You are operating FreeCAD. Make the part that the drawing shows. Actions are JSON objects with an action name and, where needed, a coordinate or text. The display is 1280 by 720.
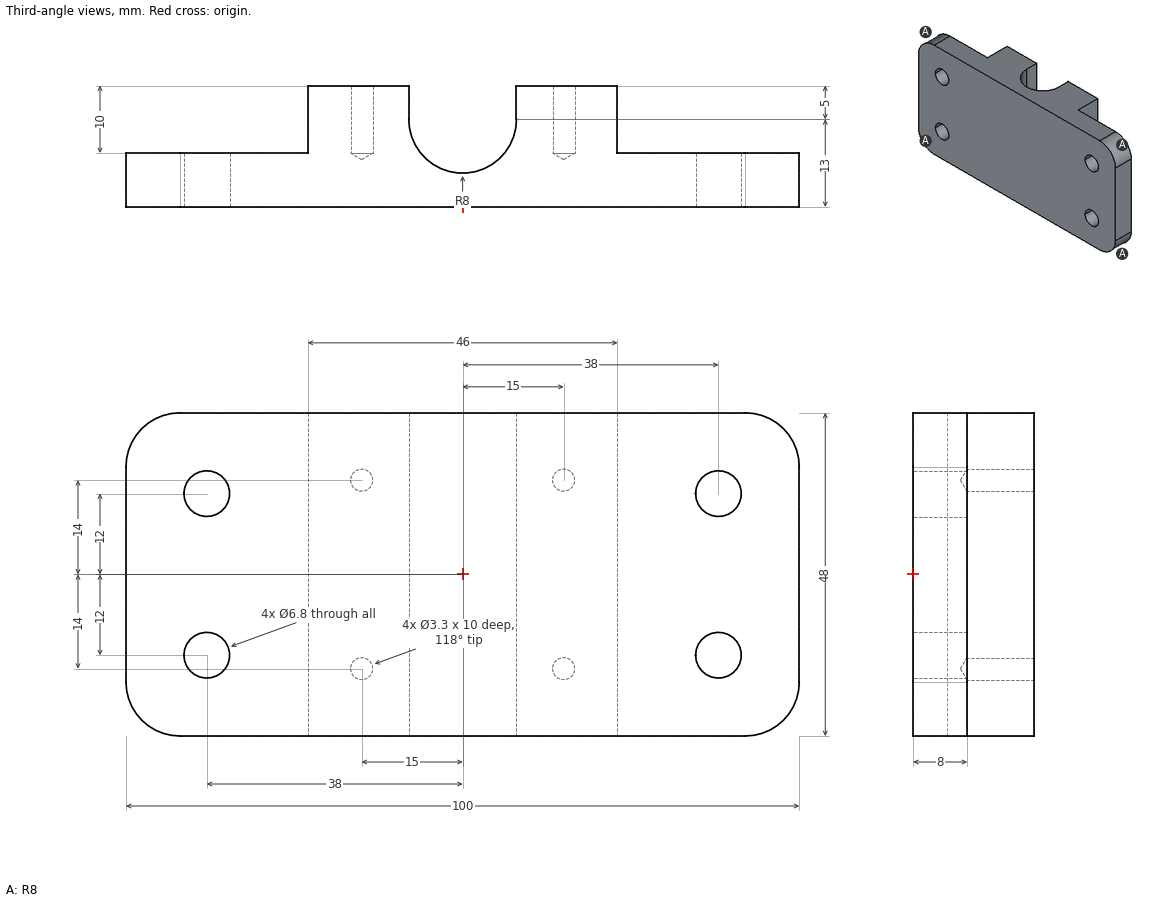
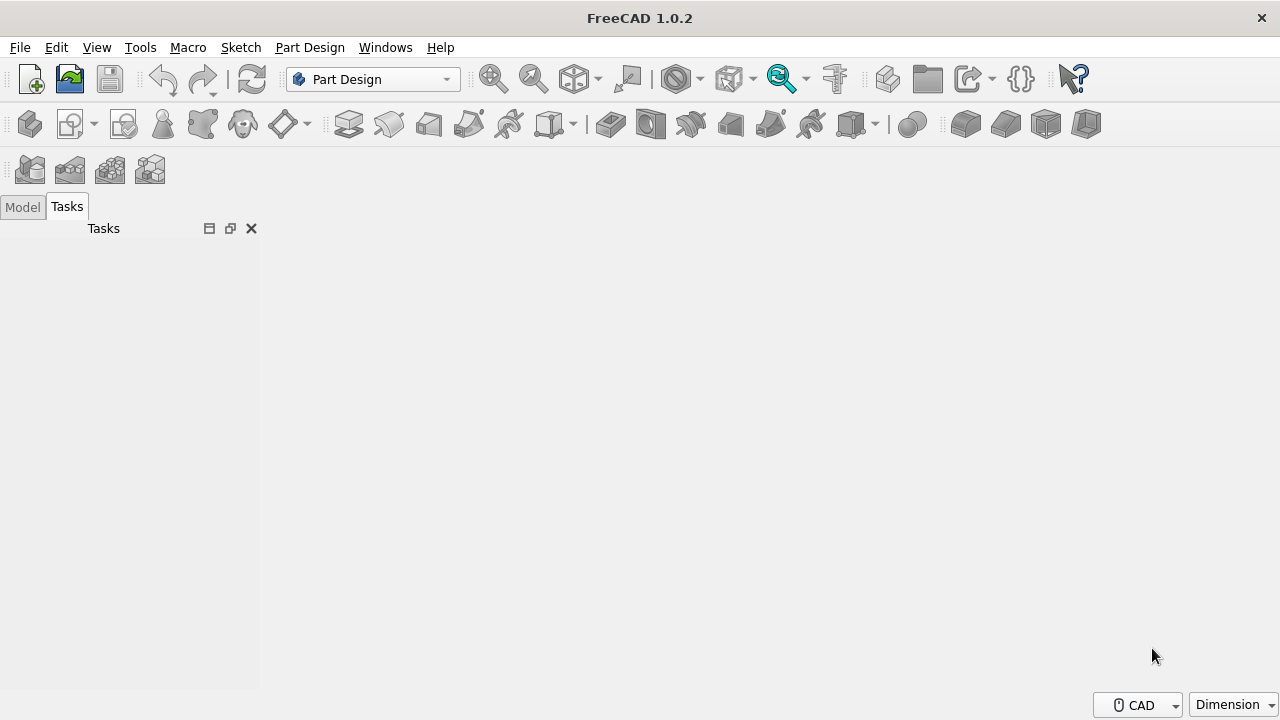
{"action": "left_click", "coordinate": [30, 80]}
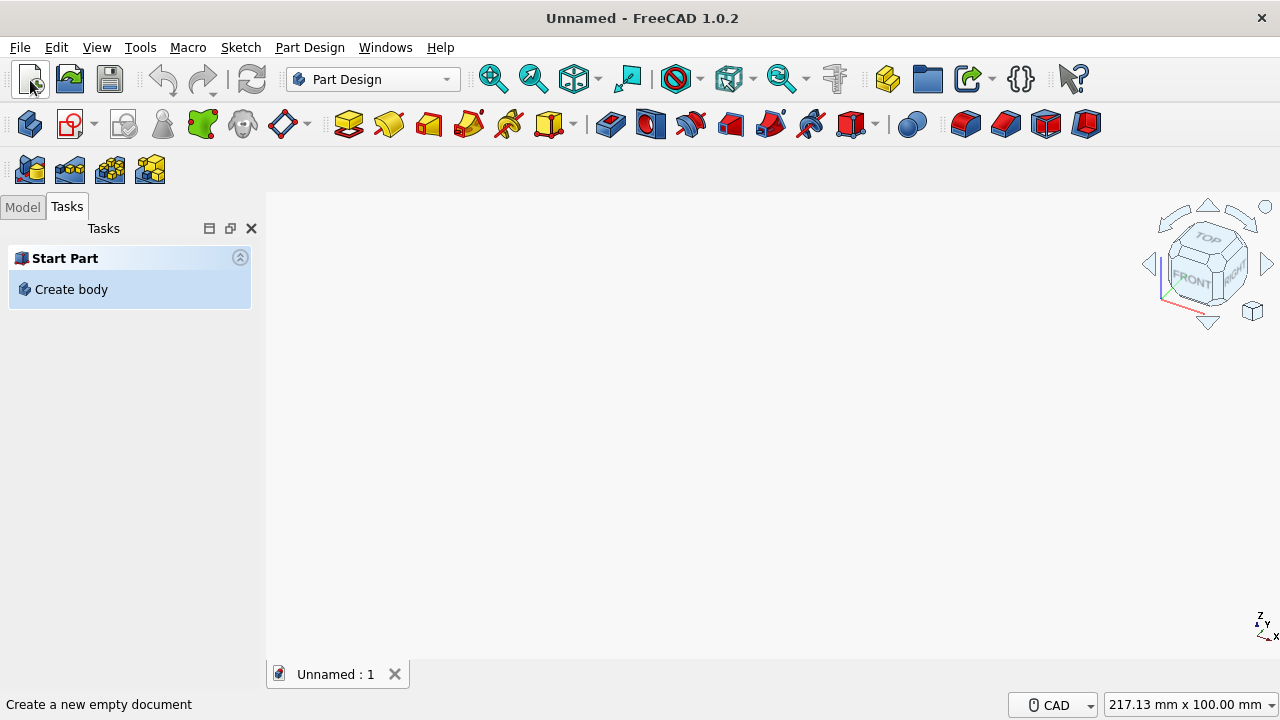
{"action": "left_click", "coordinate": [70, 124]}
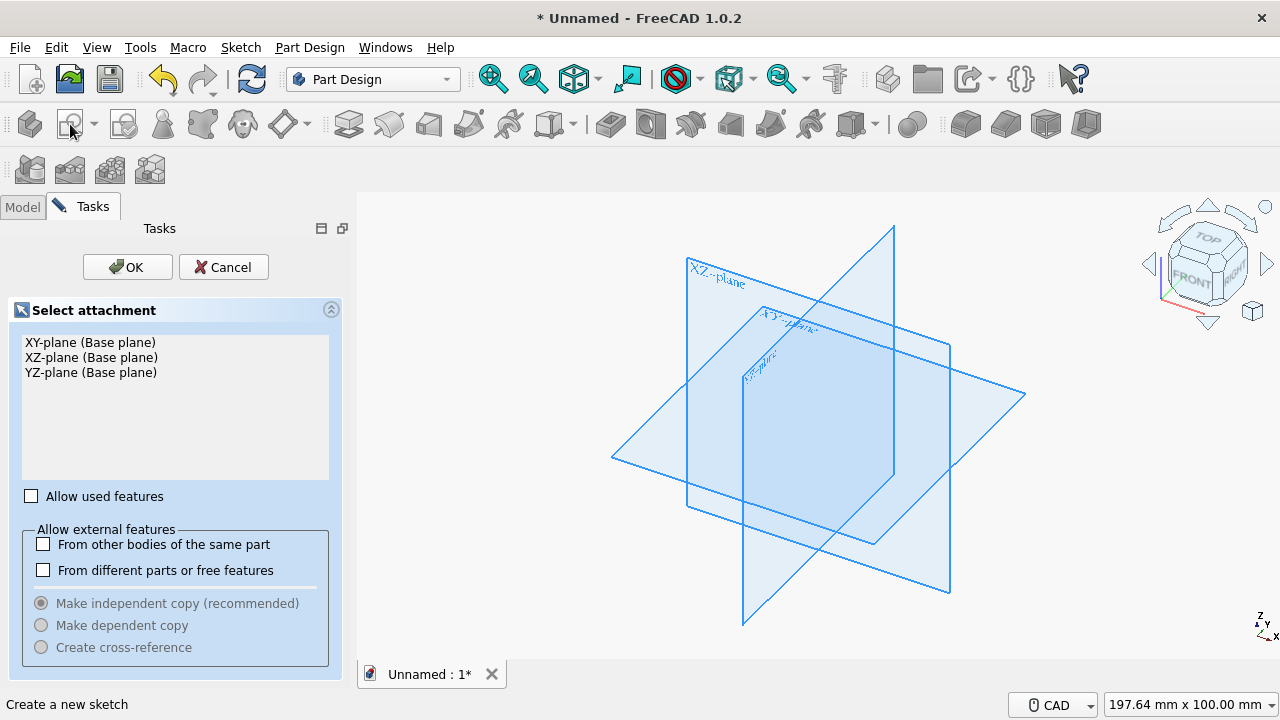
{"action": "left_click", "coordinate": [82, 358]}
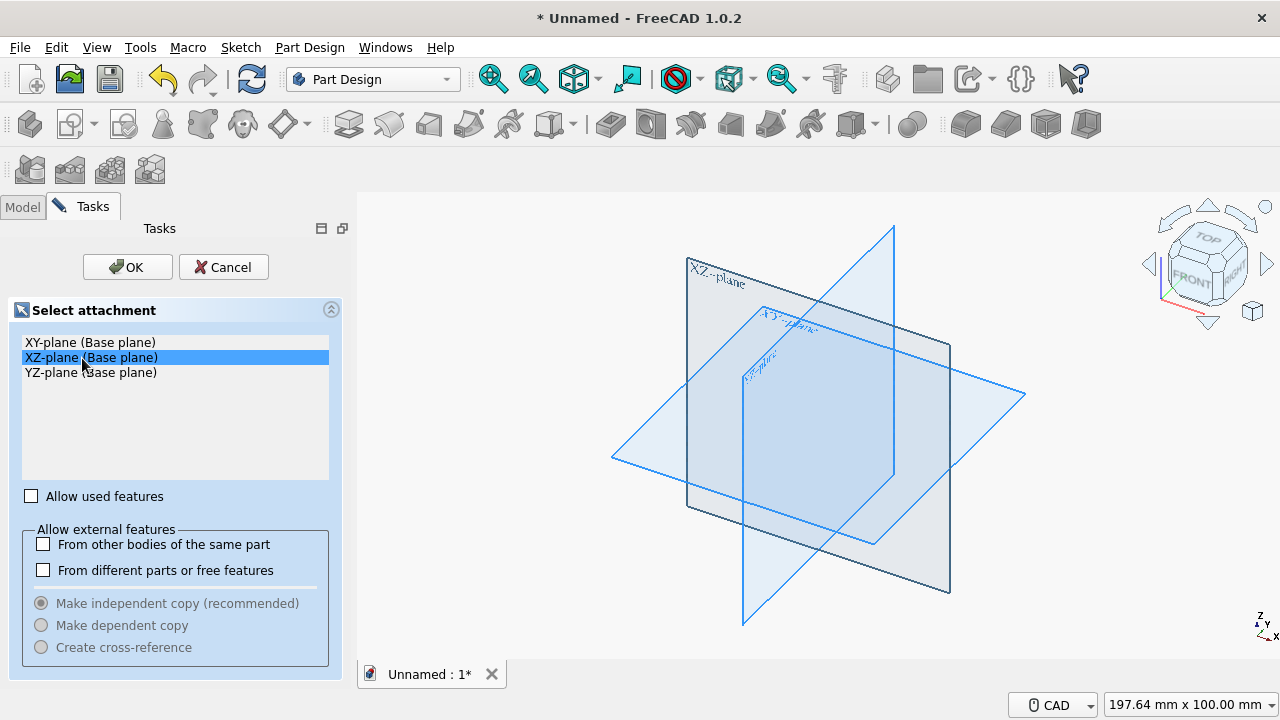
{"action": "left_click", "coordinate": [128, 267]}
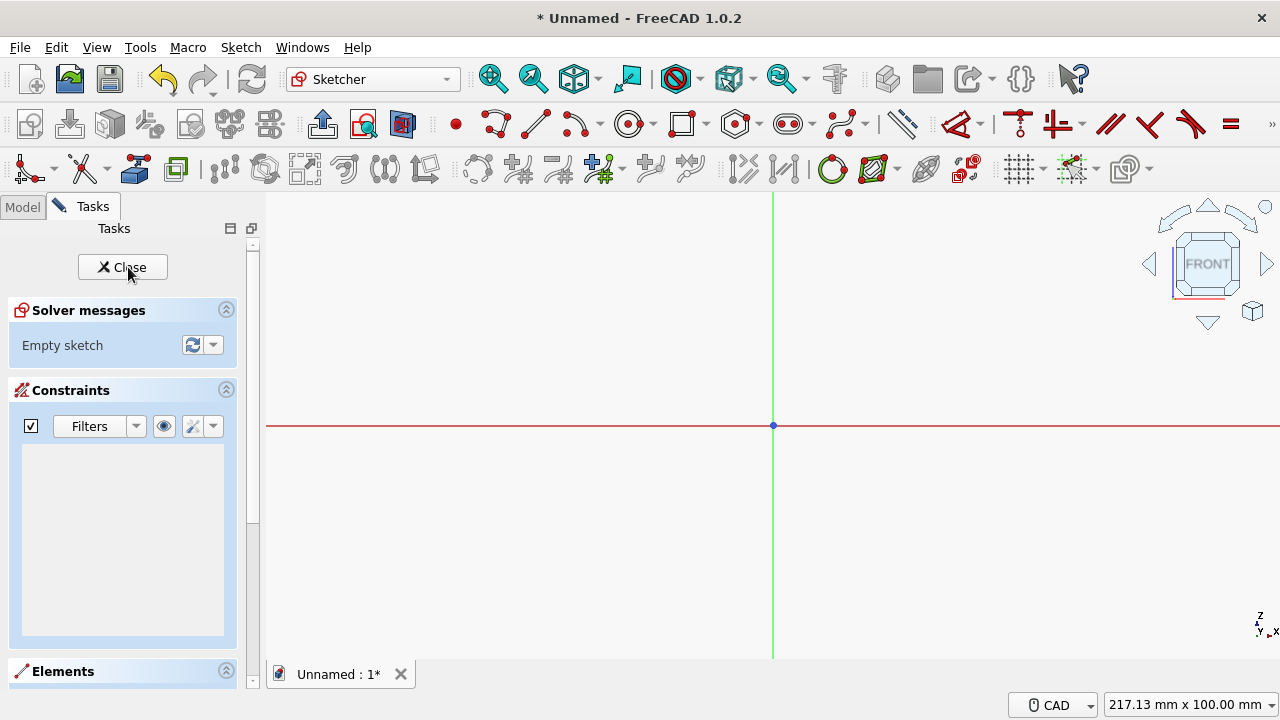
{"action": "key", "text": "g v"}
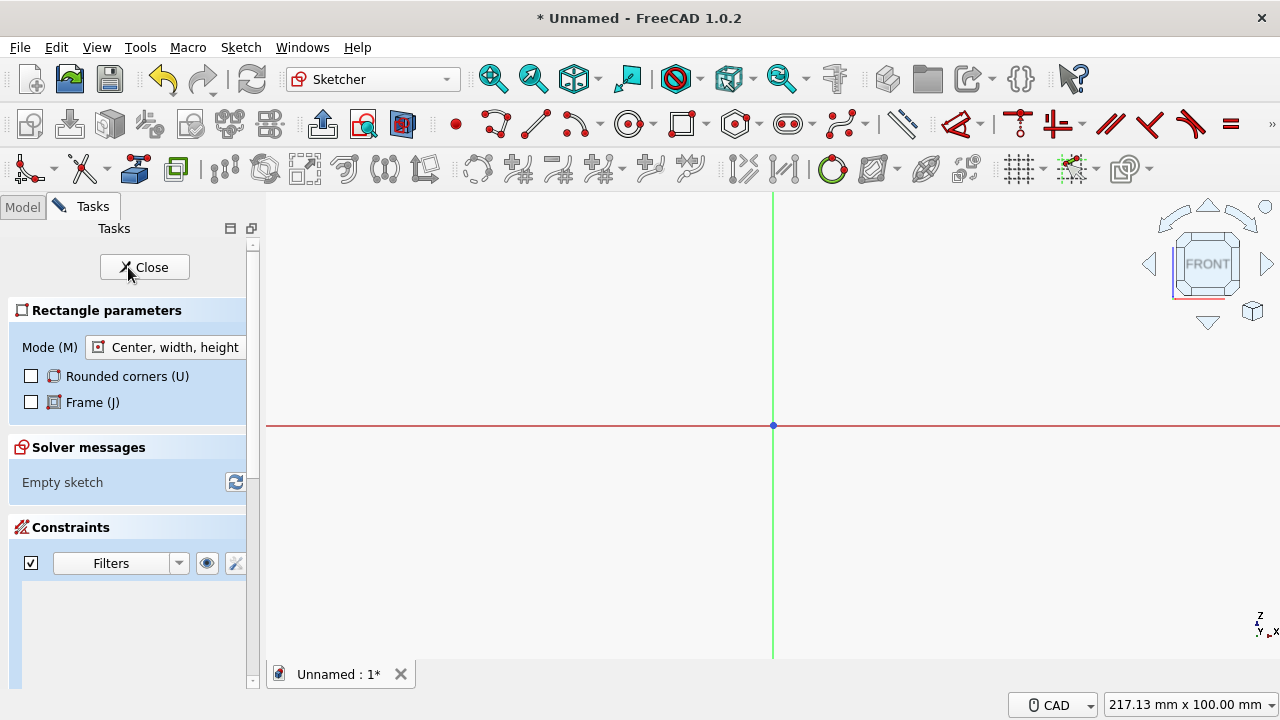
{"action": "left_click", "coordinate": [773, 426]}
{"action": "left_click", "coordinate": [1006, 313]}
{"action": "key", "text": "Escape"}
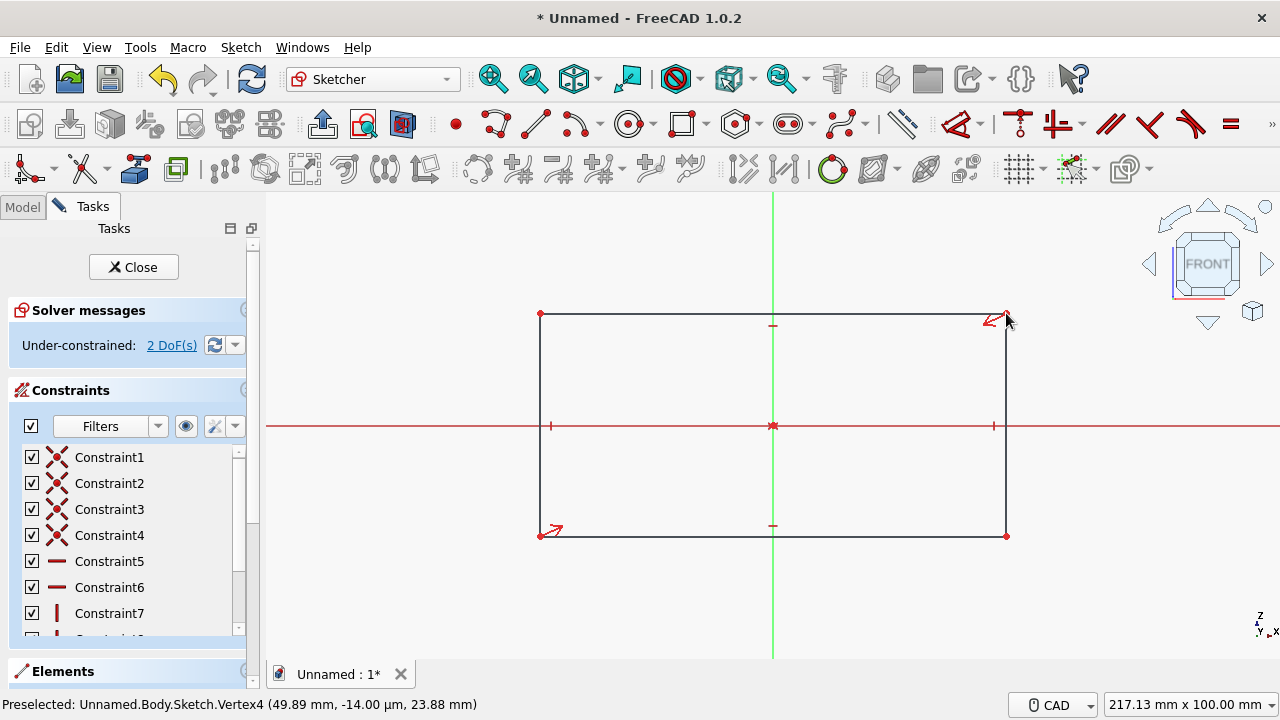
{"action": "left_click", "coordinate": [1006, 470]}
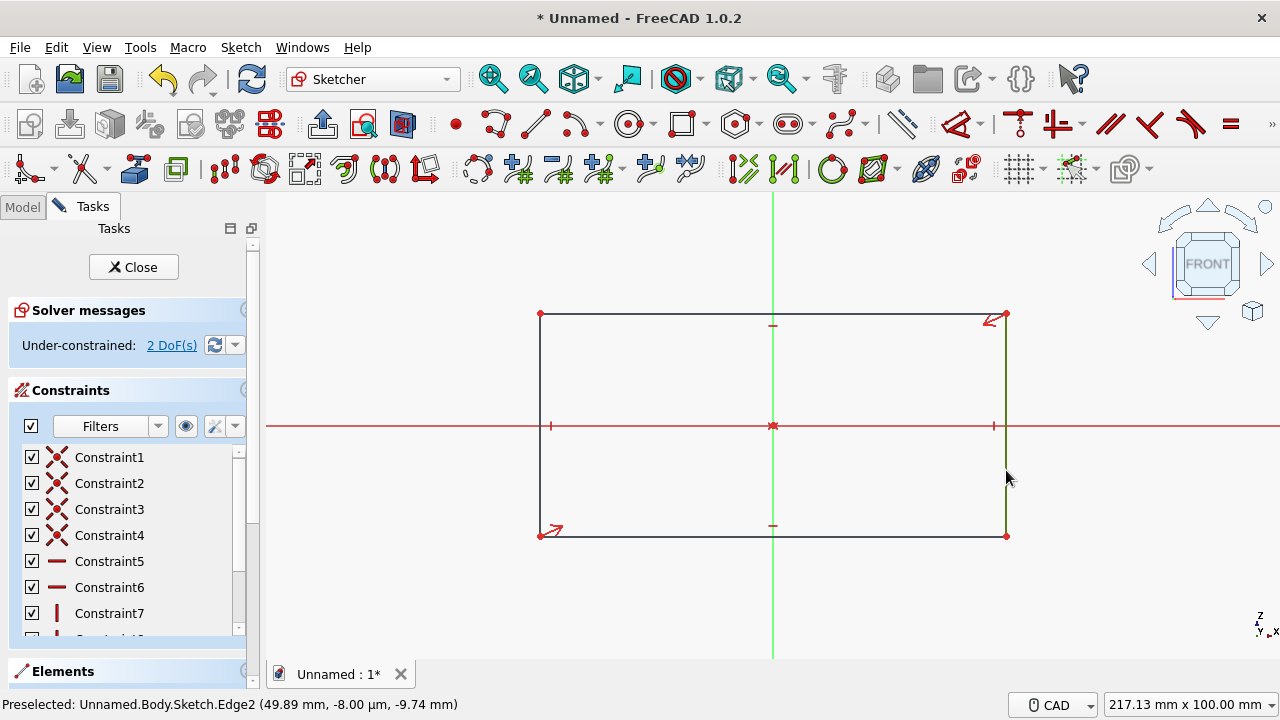
{"action": "key", "text": "i"}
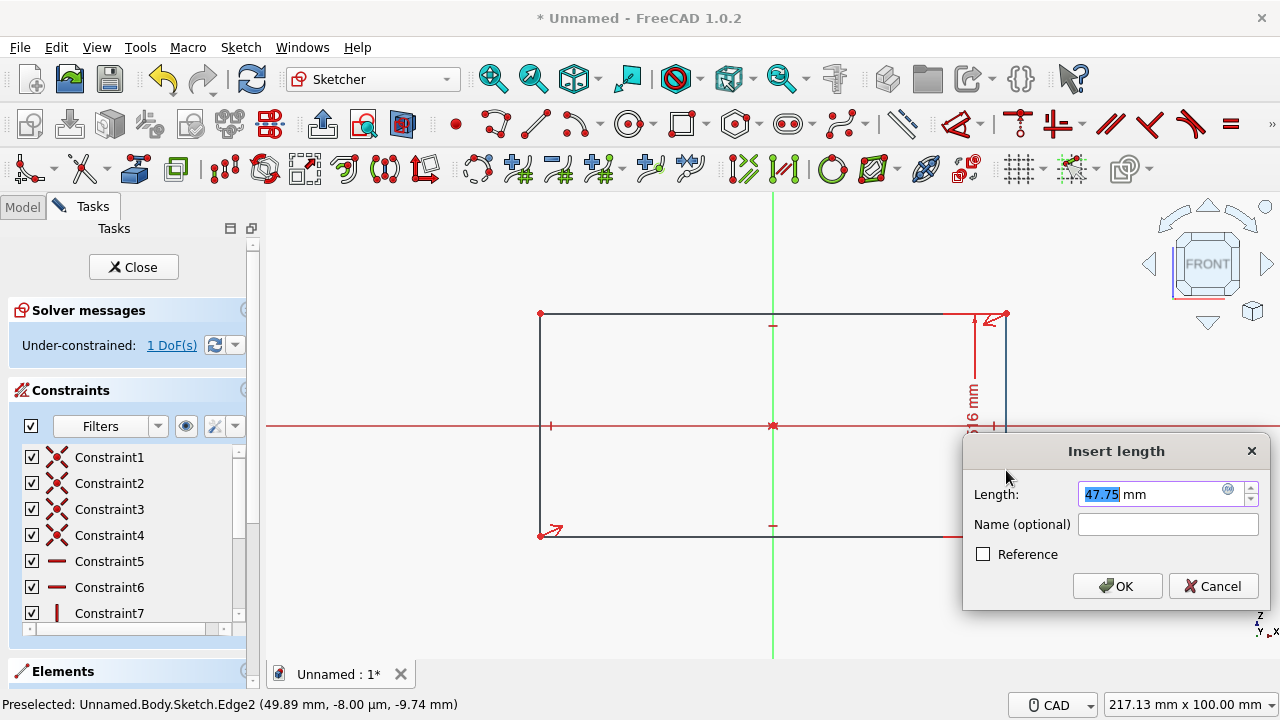
{"action": "type", "text": "48"}
{"action": "key", "text": "Return"}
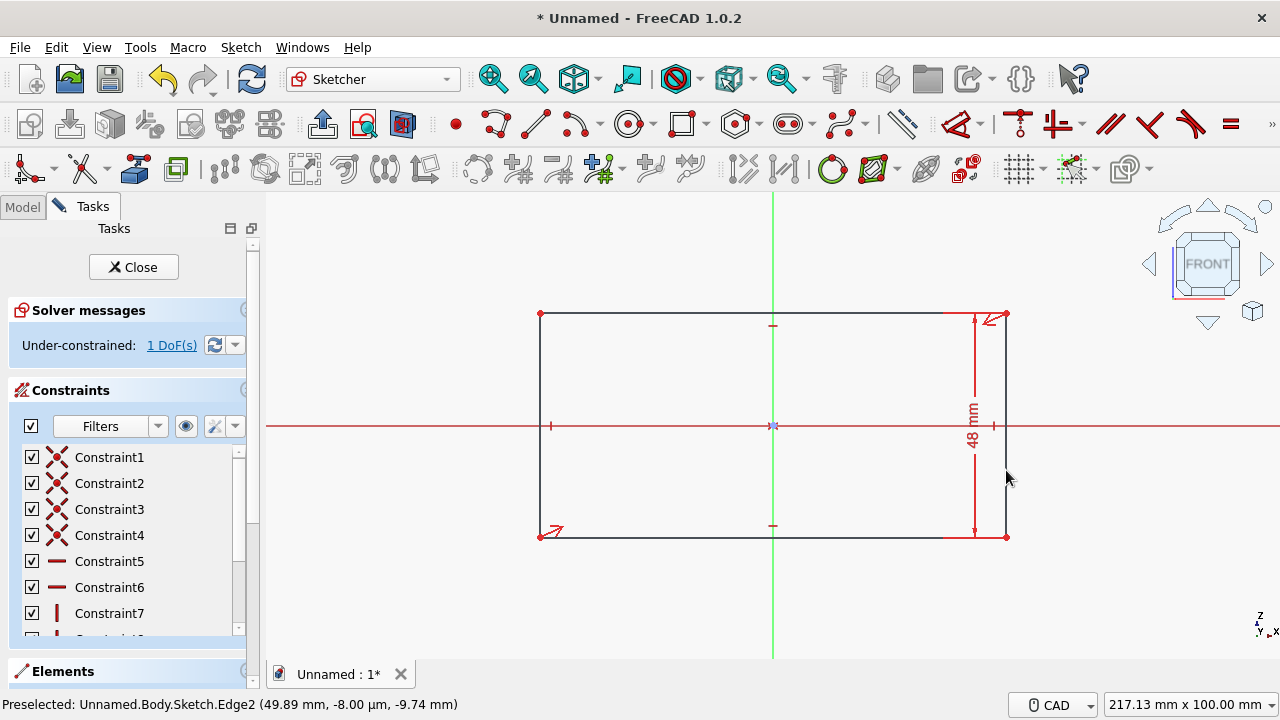
{"action": "left_click", "coordinate": [680, 538]}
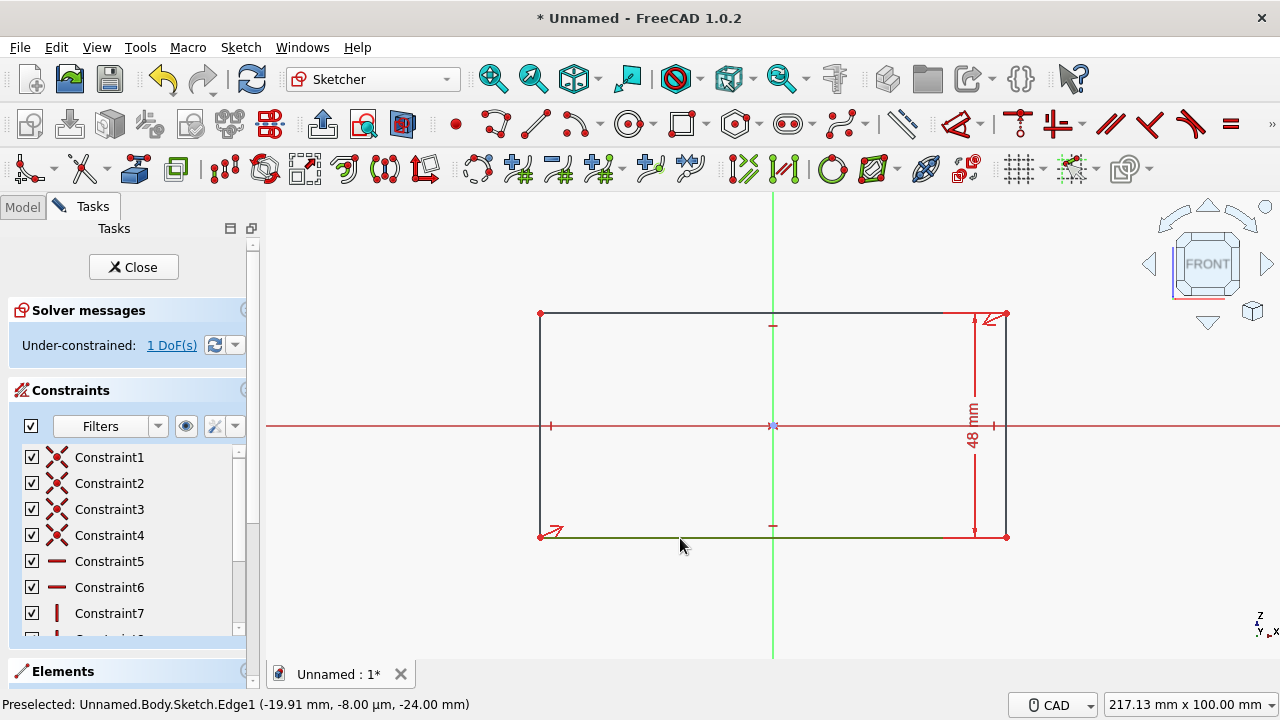
{"action": "left_click", "coordinate": [982, 124]}